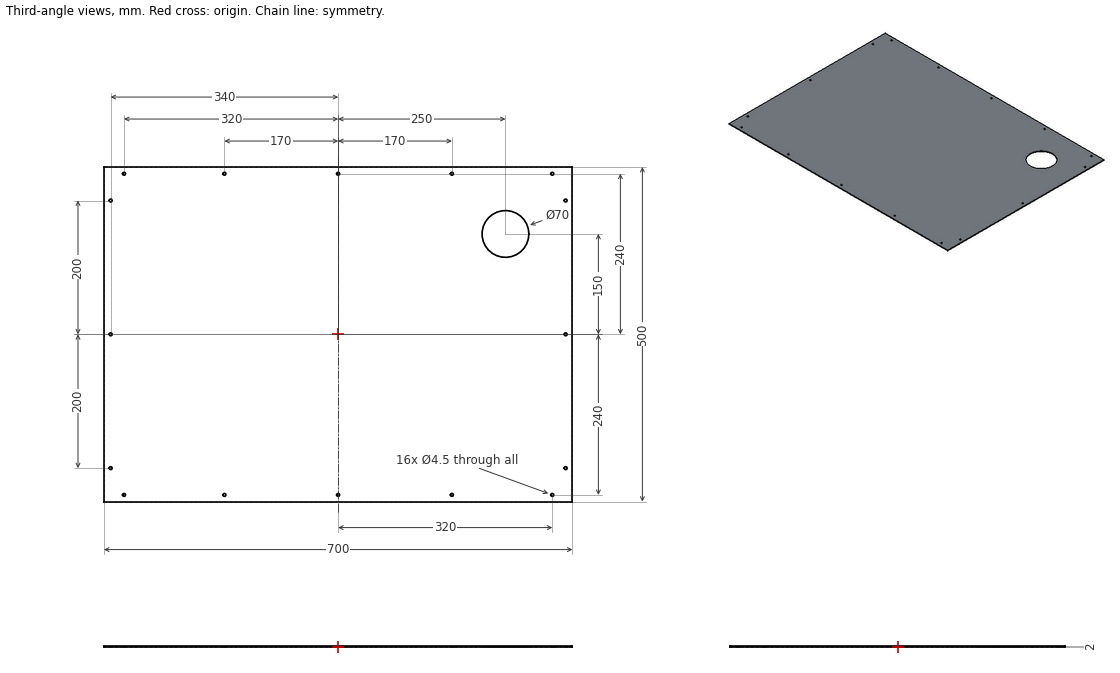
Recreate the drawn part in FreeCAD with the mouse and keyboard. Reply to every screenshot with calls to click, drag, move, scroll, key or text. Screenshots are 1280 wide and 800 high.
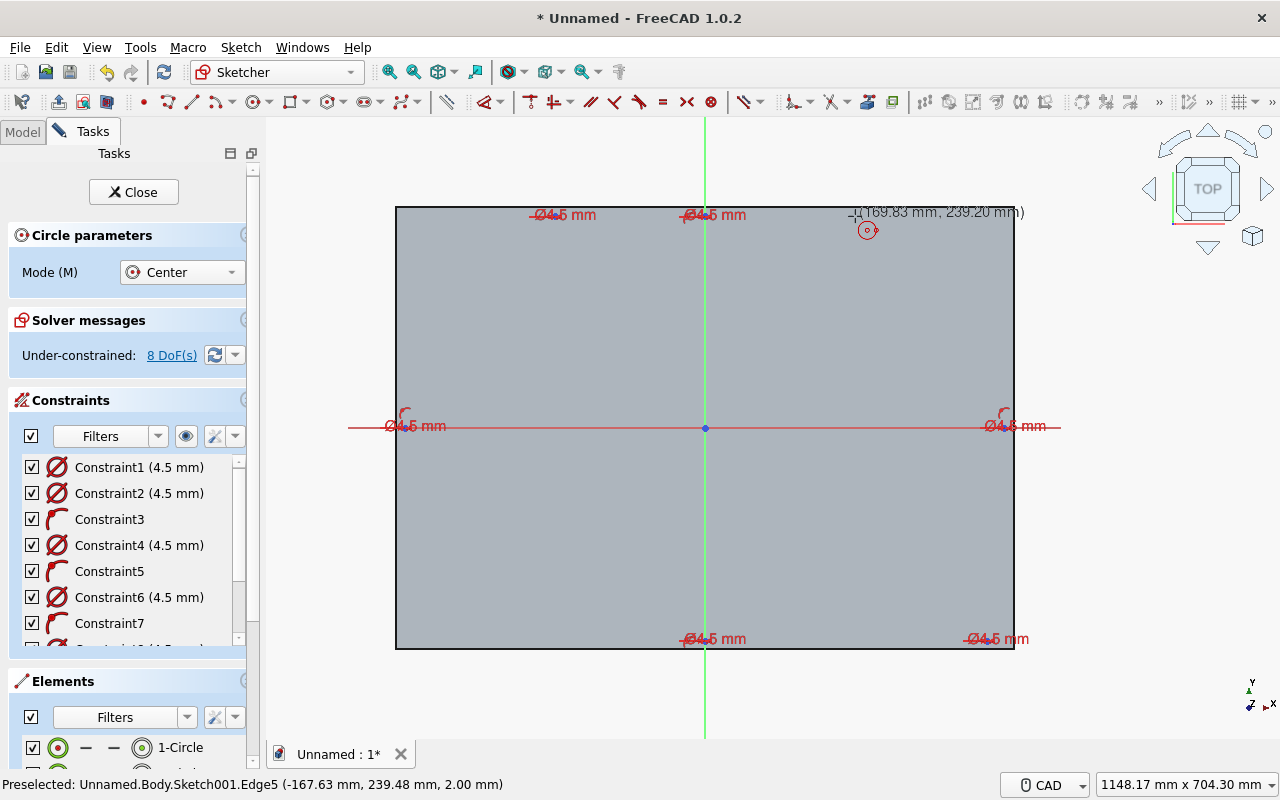
click(855, 216)
move(857, 215)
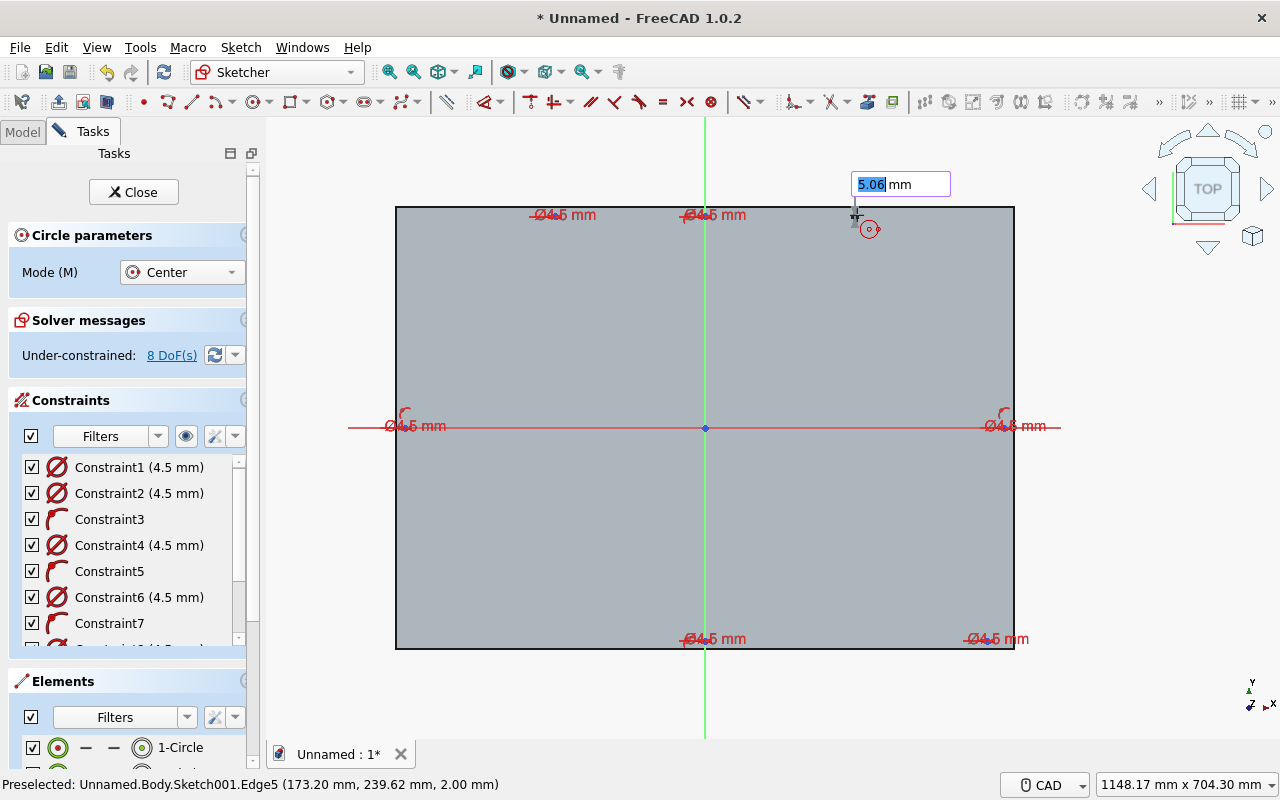
text(4.5)
key(Return)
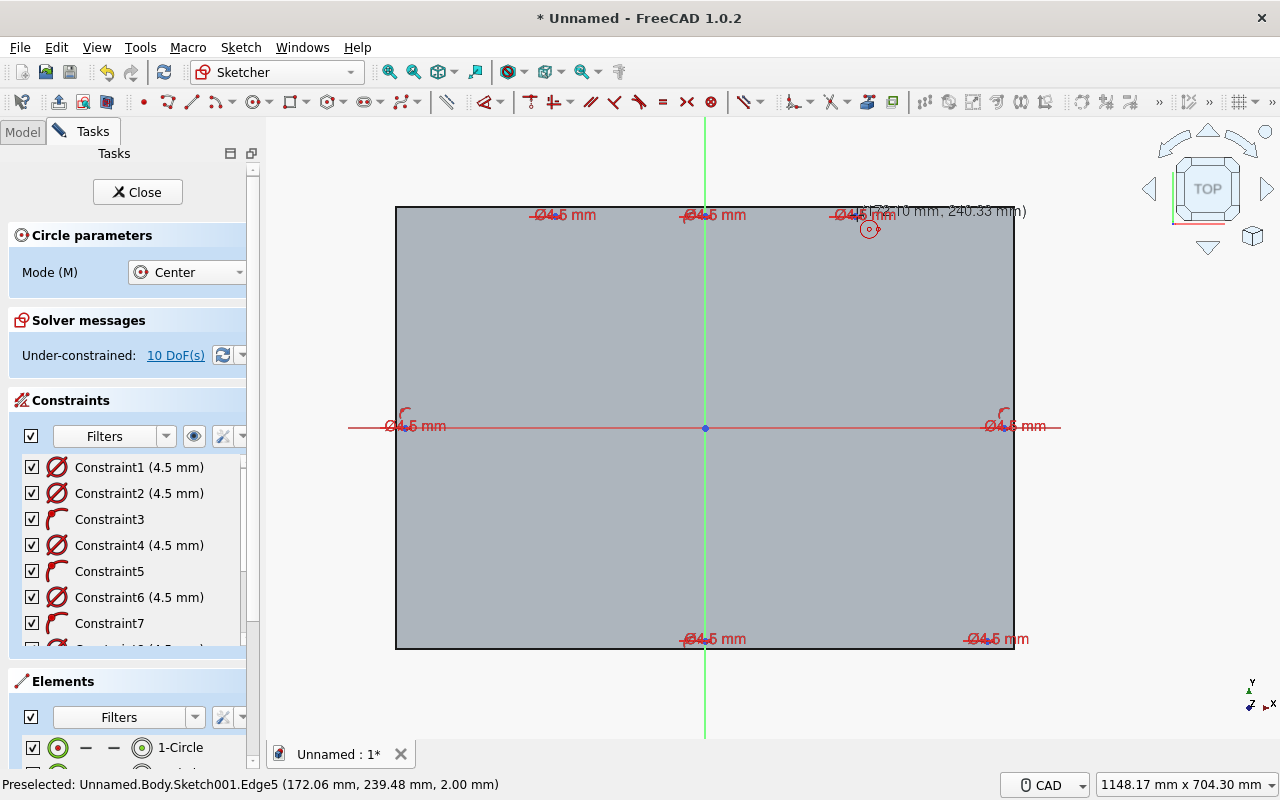
scroll(555, 640, up, 13)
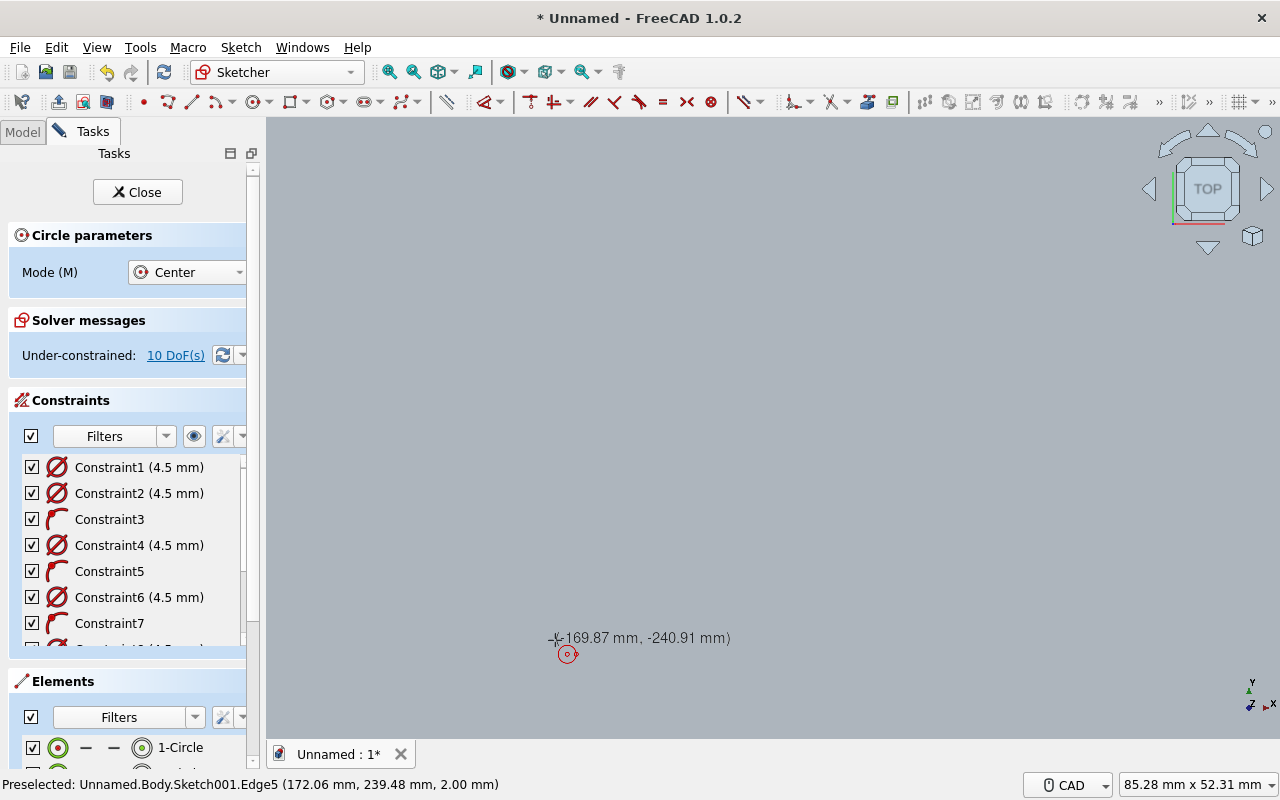
scroll(555, 641, down, 13)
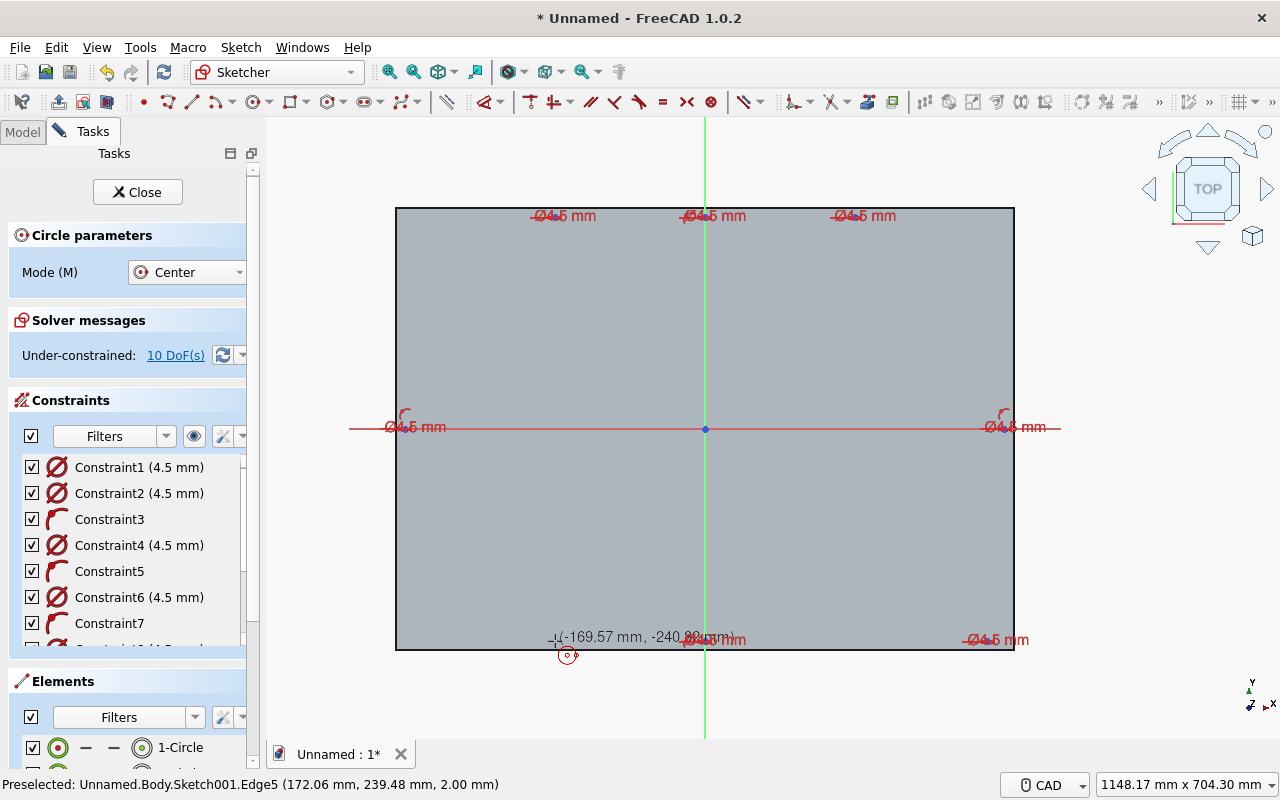
click(555, 641)
move(556, 640)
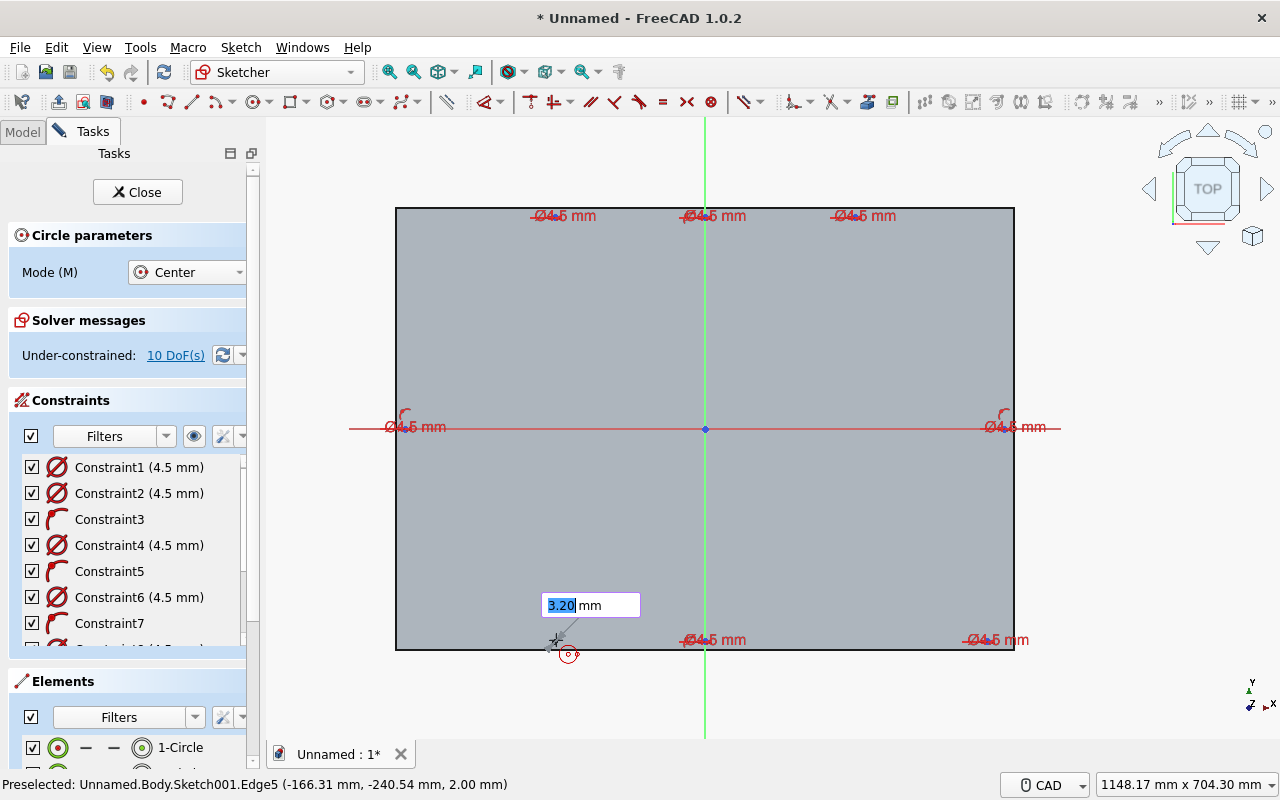
text(4.5)
key(Return)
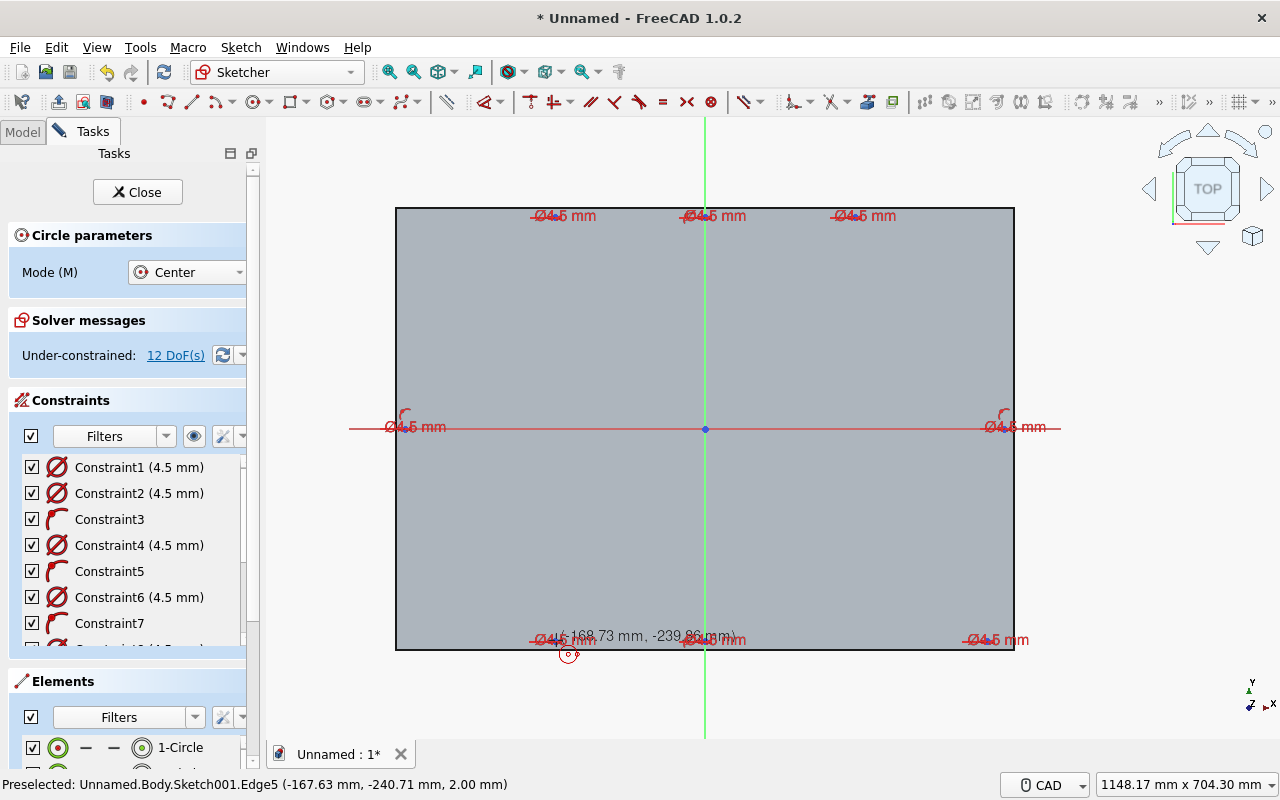
scroll(855, 641, up, 13)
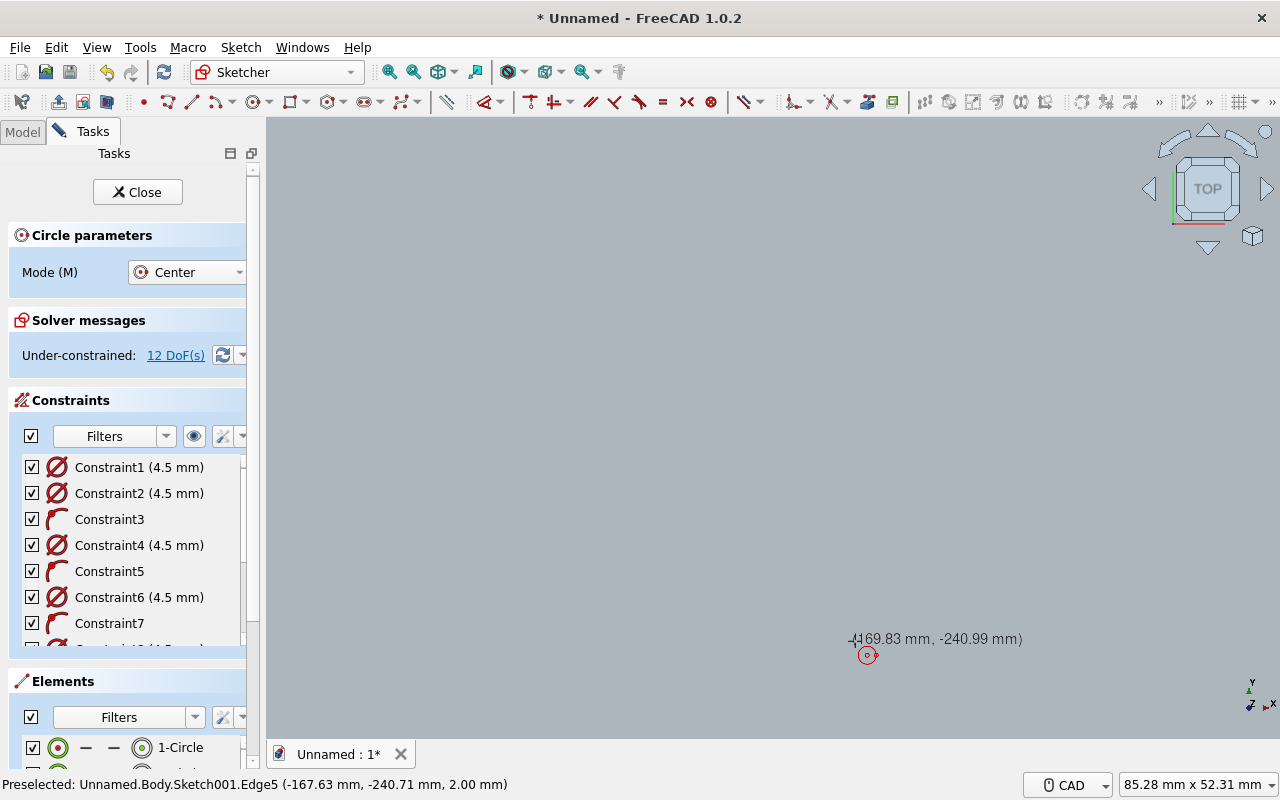
scroll(855, 641, down, 13)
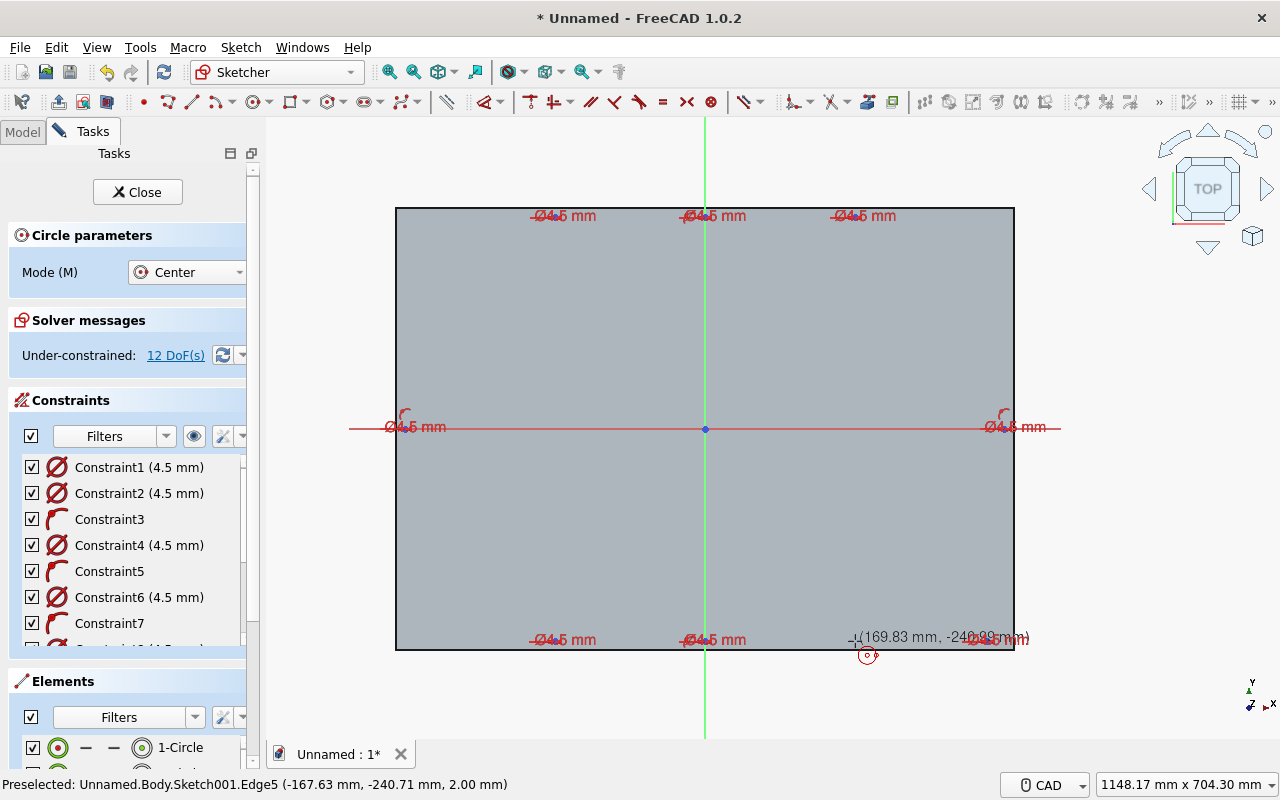
click(855, 641)
move(857, 640)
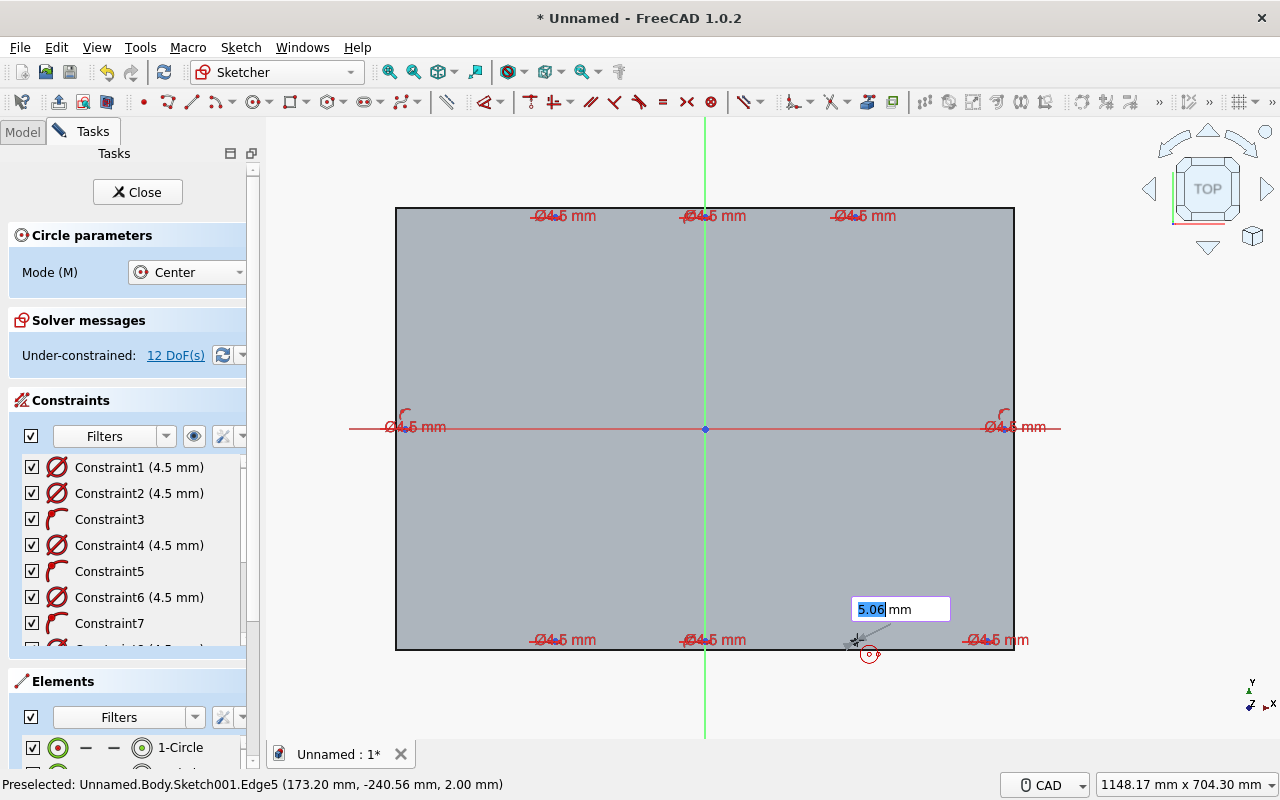
text(4.5)
key(Return)